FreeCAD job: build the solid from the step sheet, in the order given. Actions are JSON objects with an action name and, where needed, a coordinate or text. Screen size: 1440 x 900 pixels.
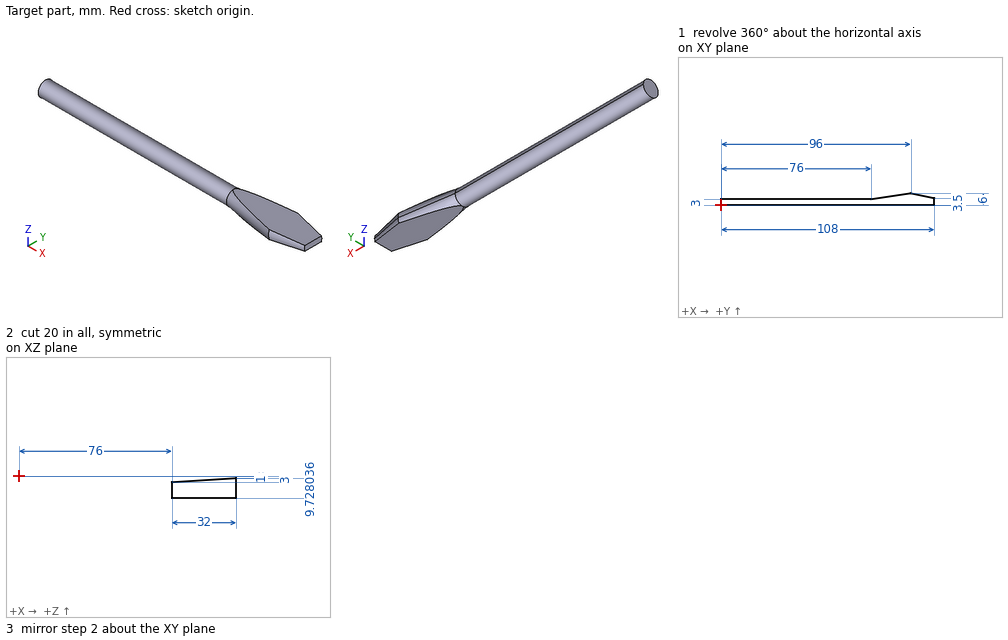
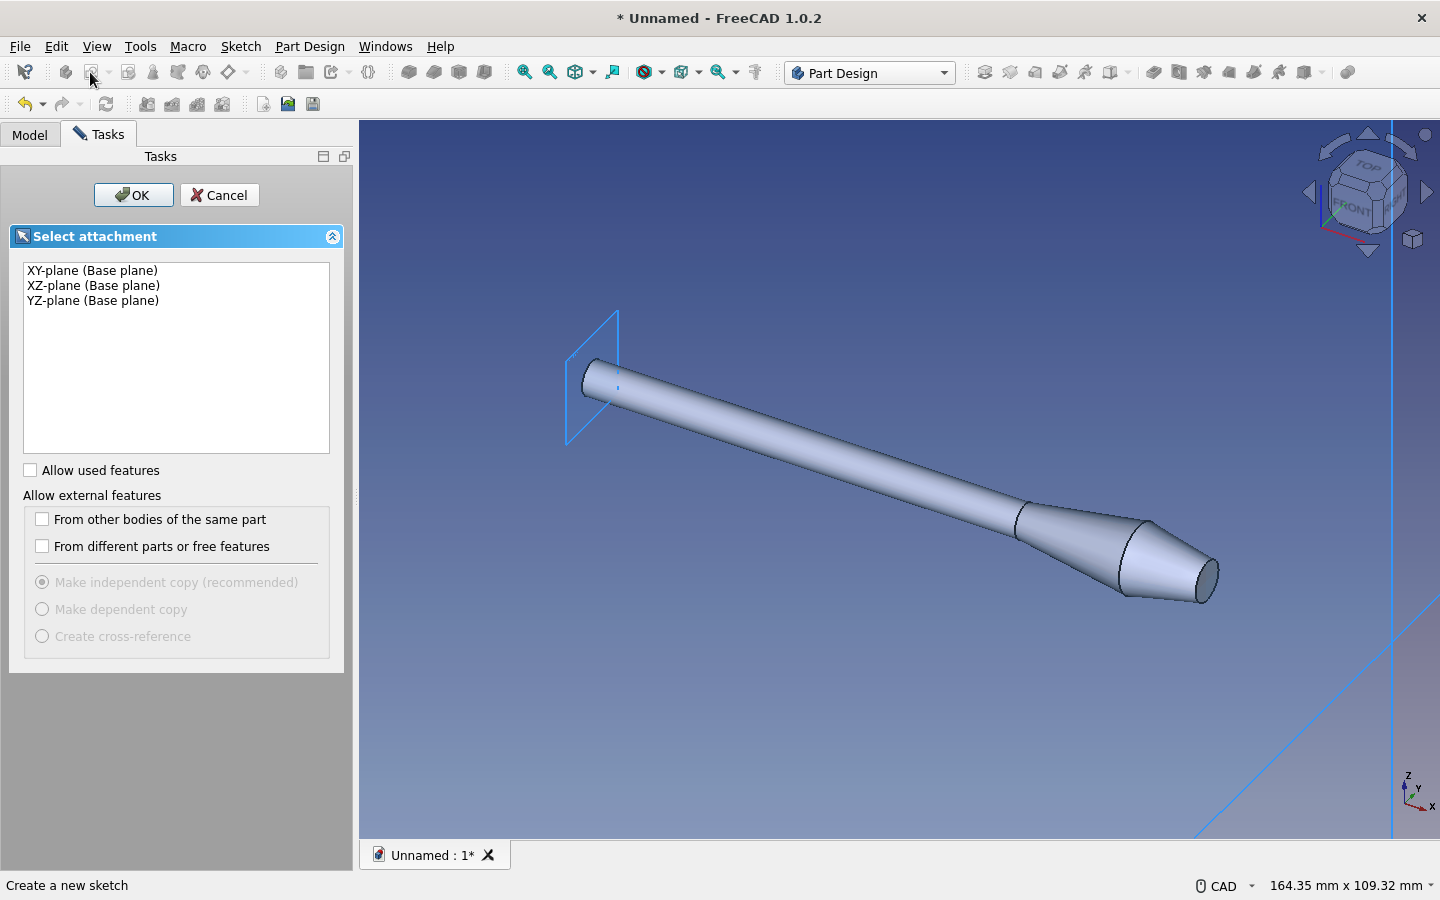
{"action": "left_click", "coordinate": [84, 286]}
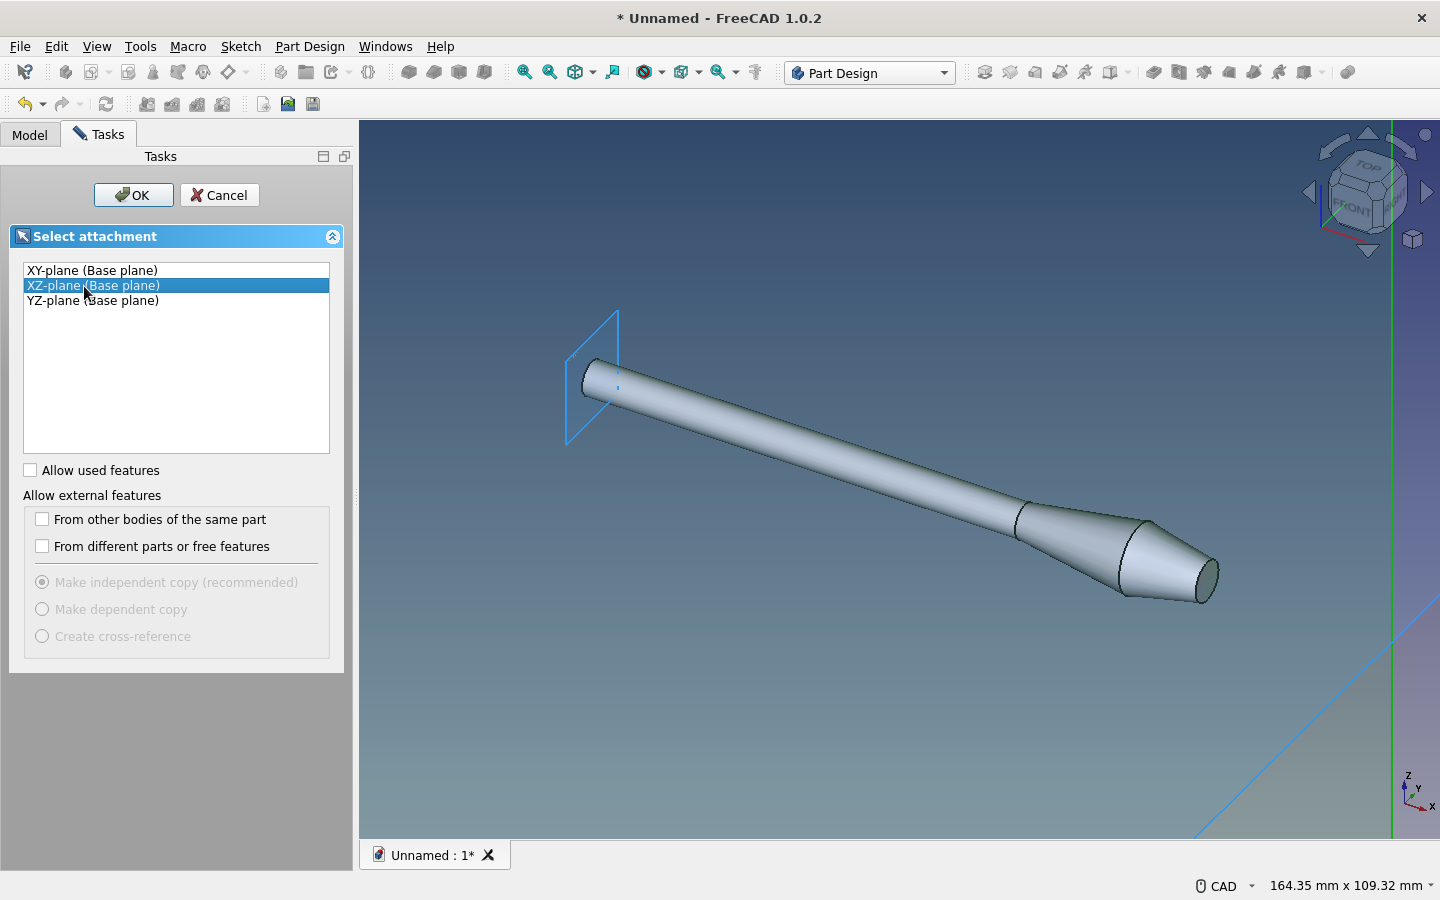
{"action": "left_click", "coordinate": [134, 195]}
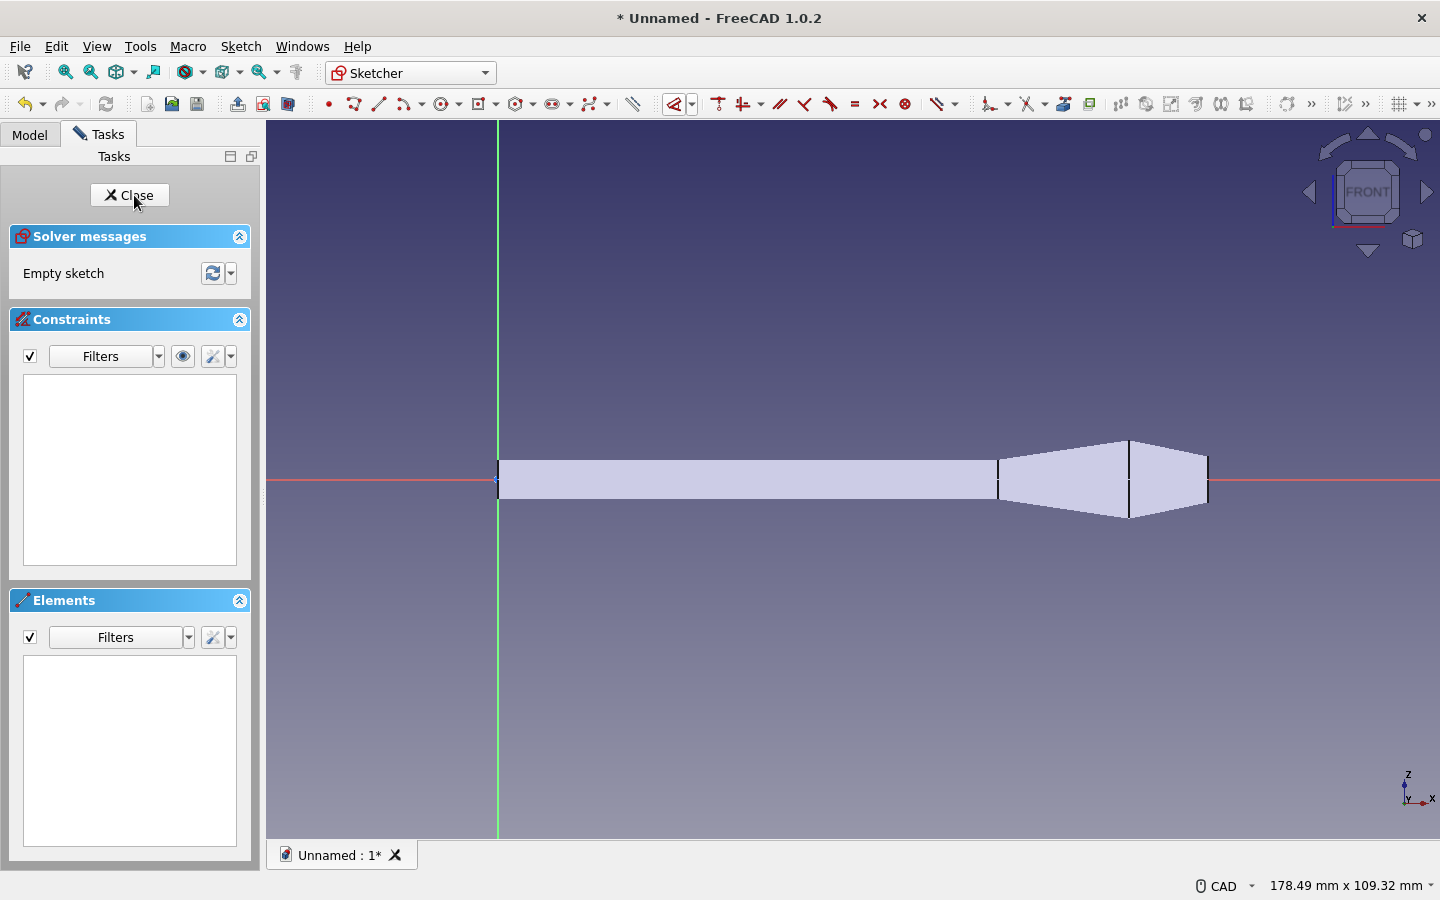
{"action": "key", "text": "q s"}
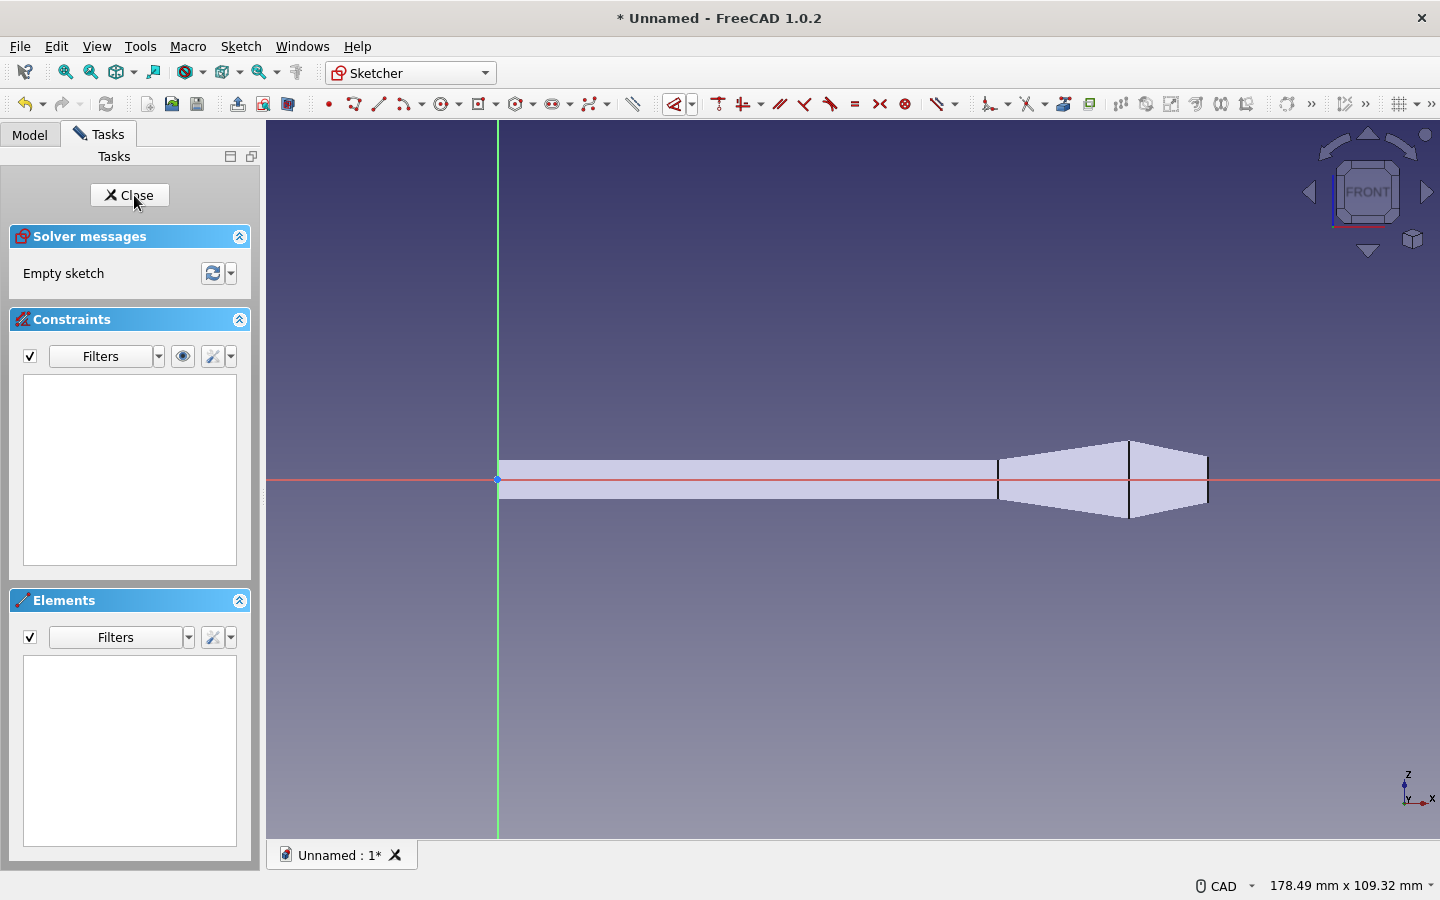
{"action": "scroll", "coordinate": [1240, 535], "scroll_direction": "up", "scroll_amount": 6}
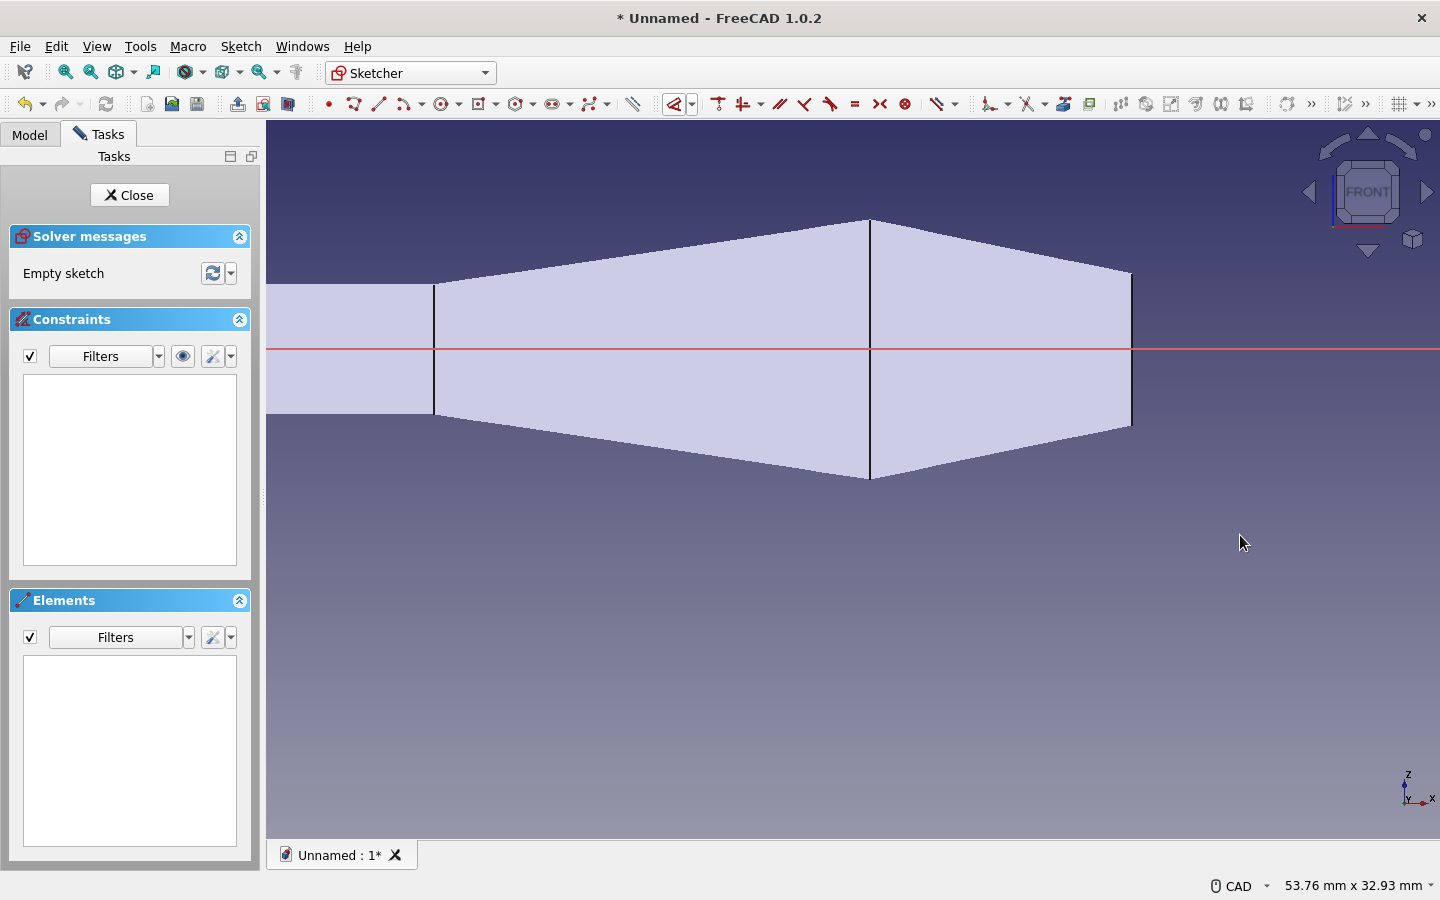
{"action": "left_click", "coordinate": [354, 104]}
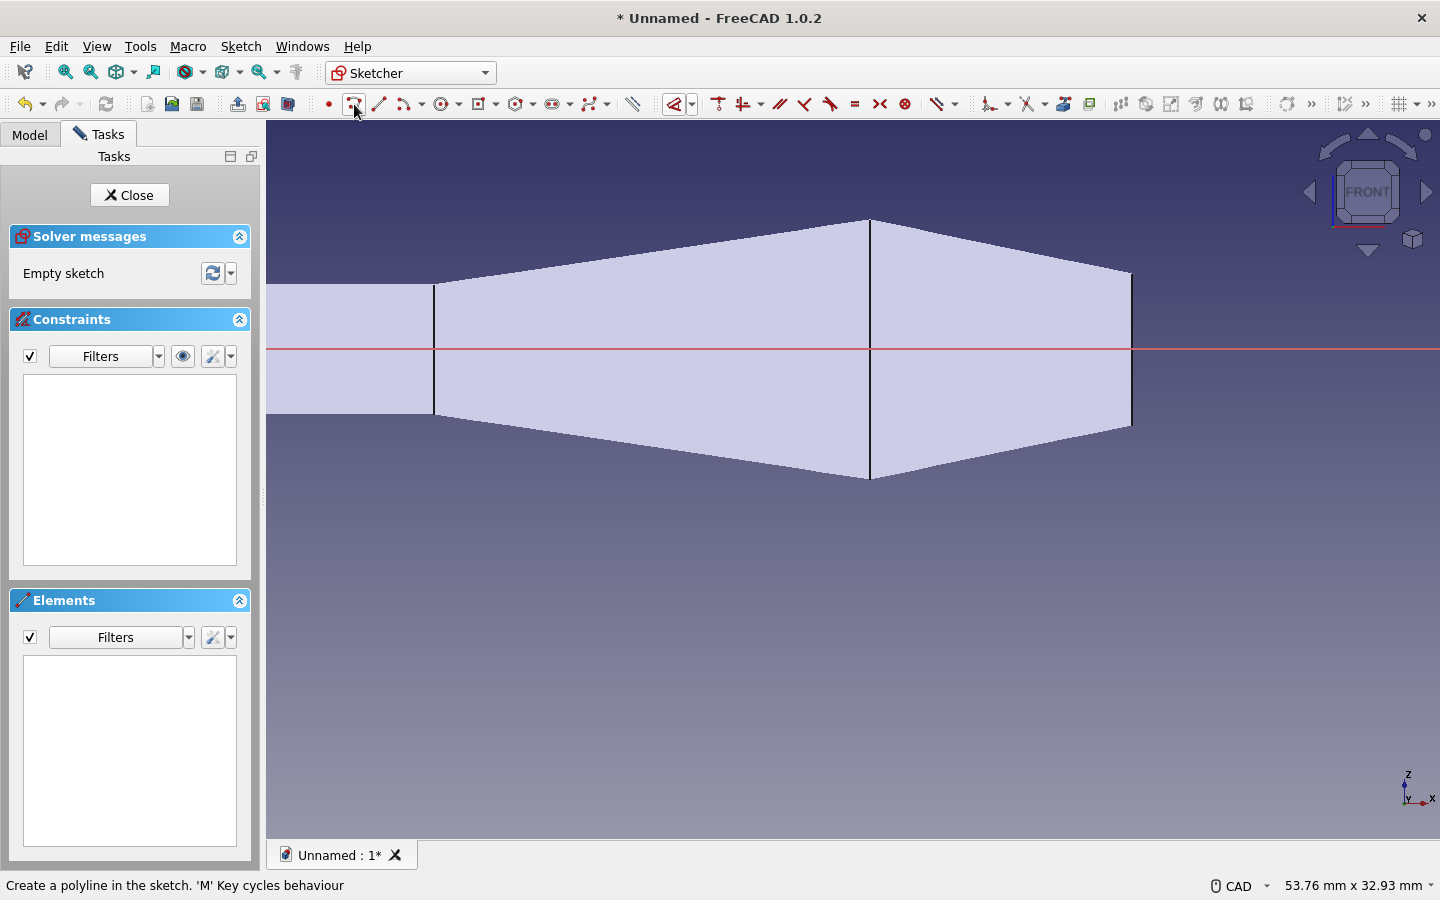
{"action": "left_click", "coordinate": [434, 415]}
{"action": "left_click", "coordinate": [1132, 371]}
{"action": "left_click", "coordinate": [1132, 584]}
{"action": "left_click", "coordinate": [434, 584]}
{"action": "left_click", "coordinate": [434, 416]}
{"action": "key", "text": "Escape"}
{"action": "key", "text": "Escape"}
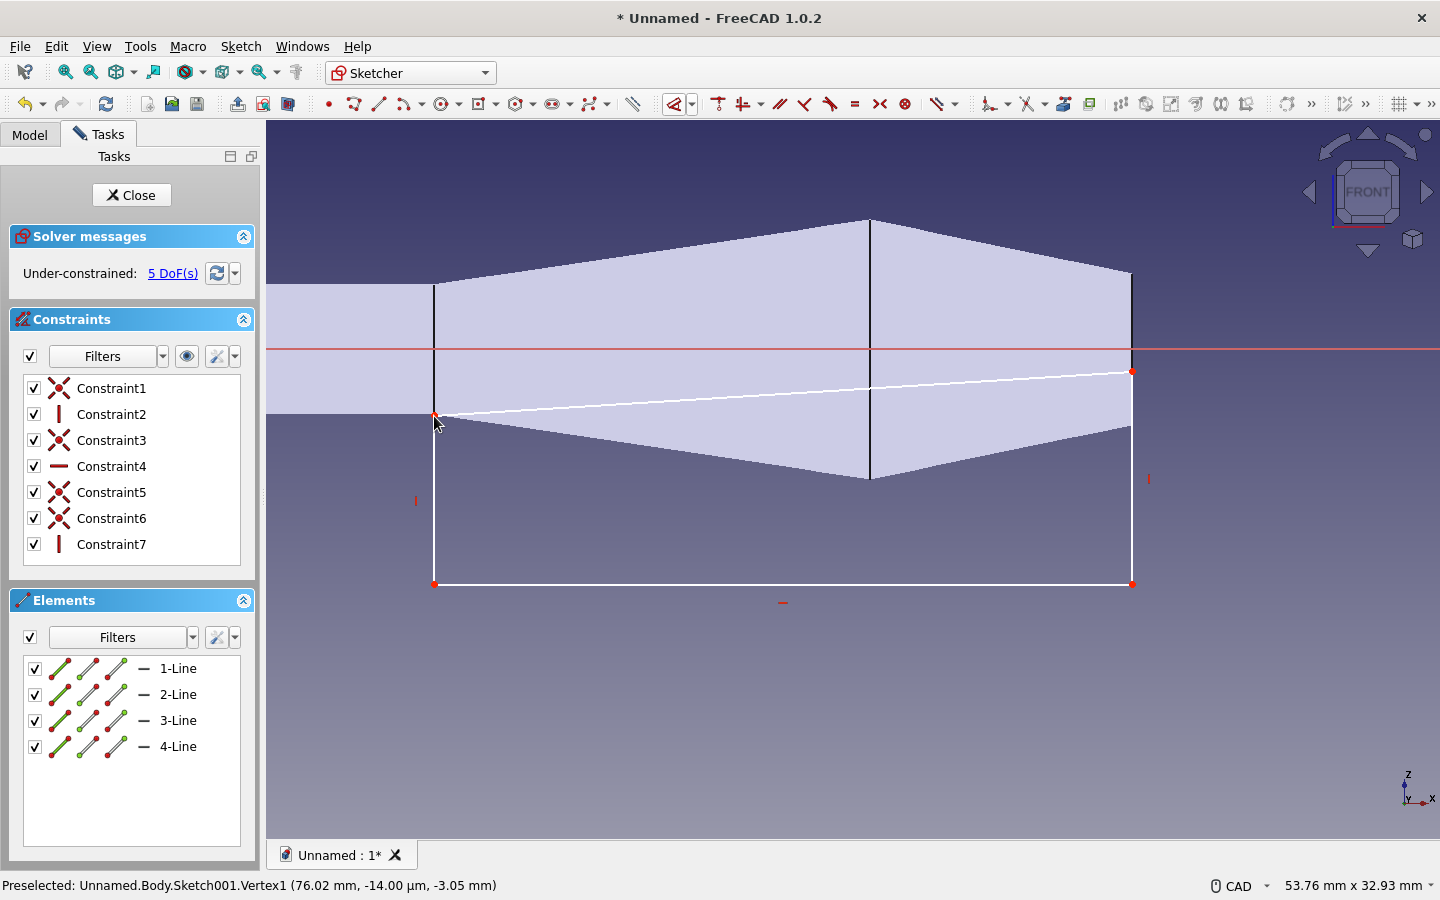
{"action": "left_click", "coordinate": [923, 585]}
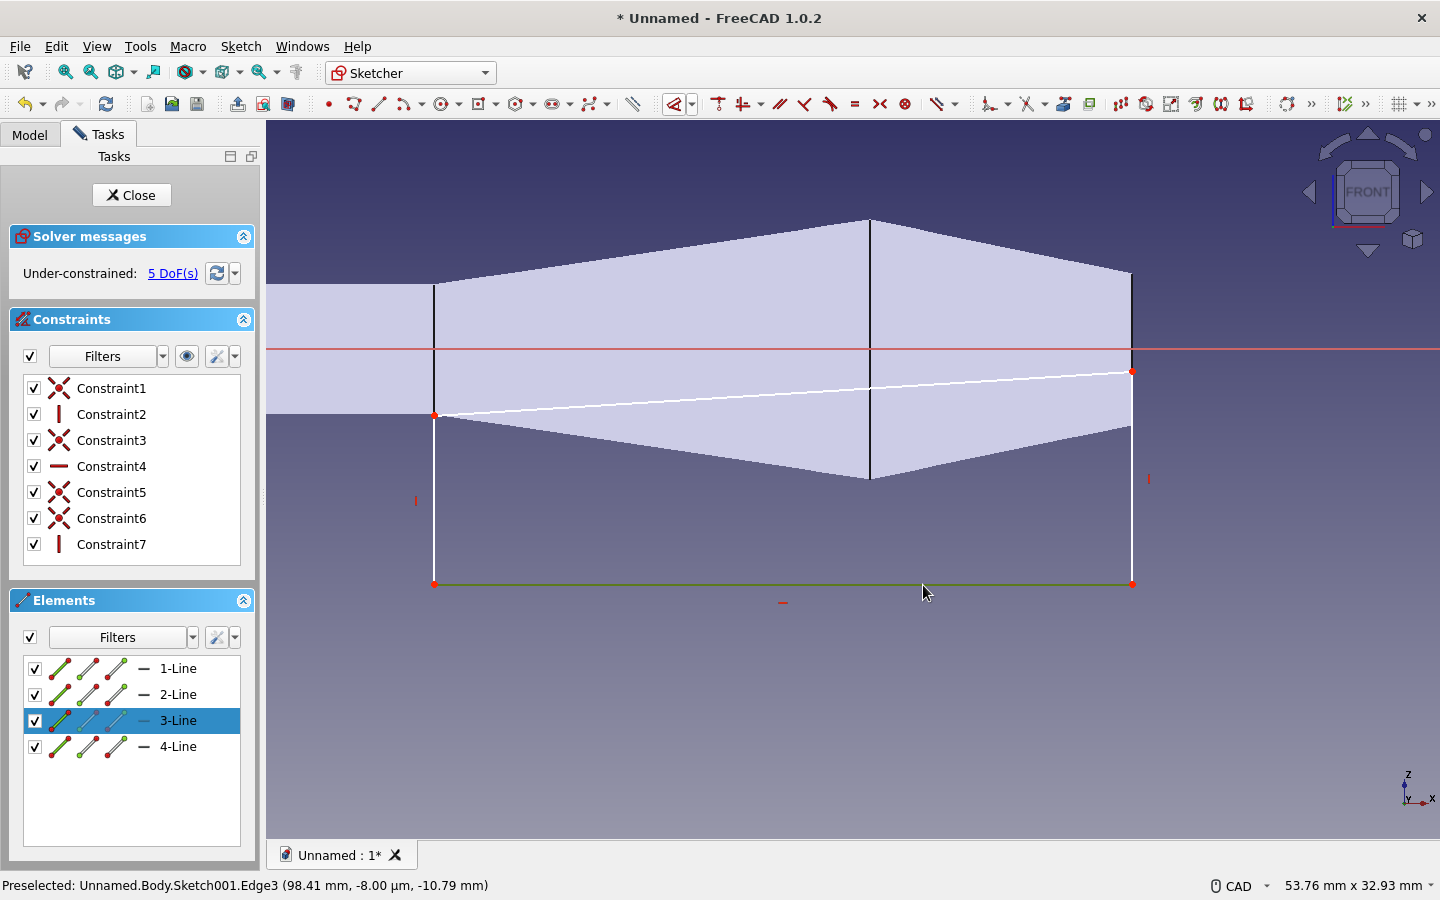
{"action": "left_click", "coordinate": [692, 104]}